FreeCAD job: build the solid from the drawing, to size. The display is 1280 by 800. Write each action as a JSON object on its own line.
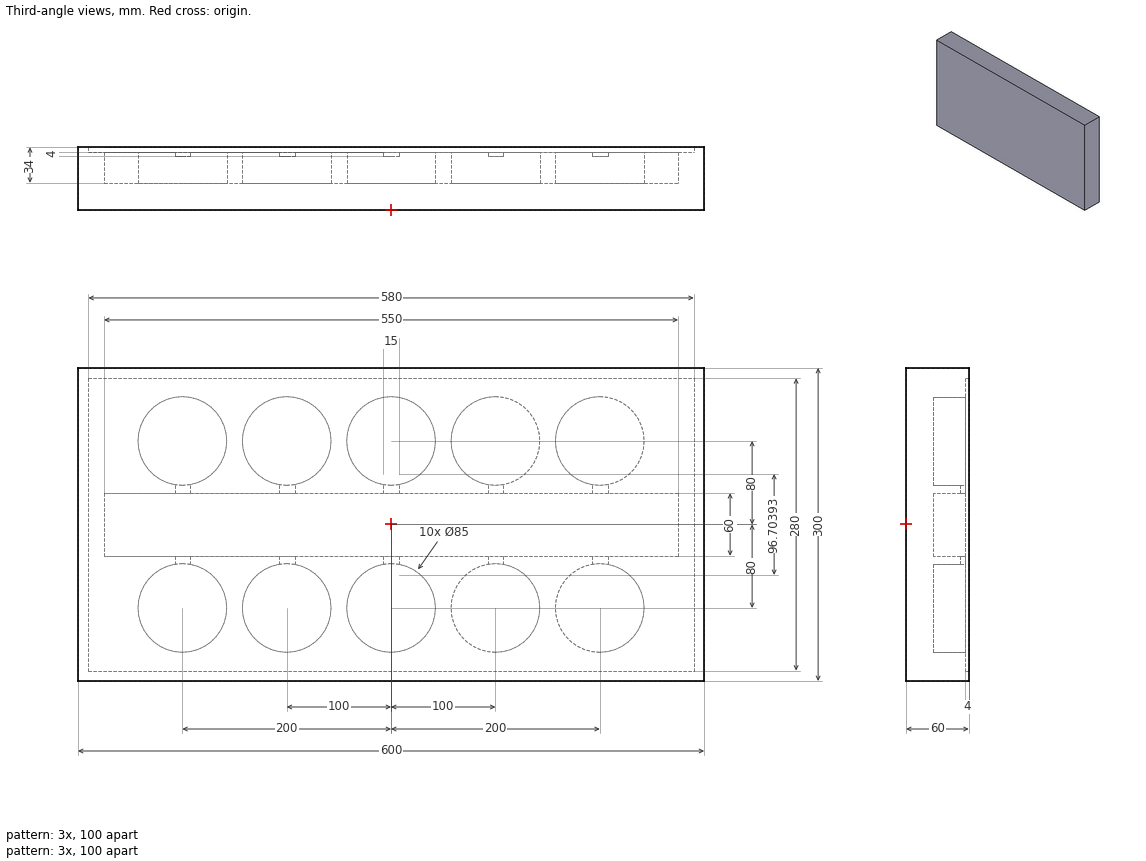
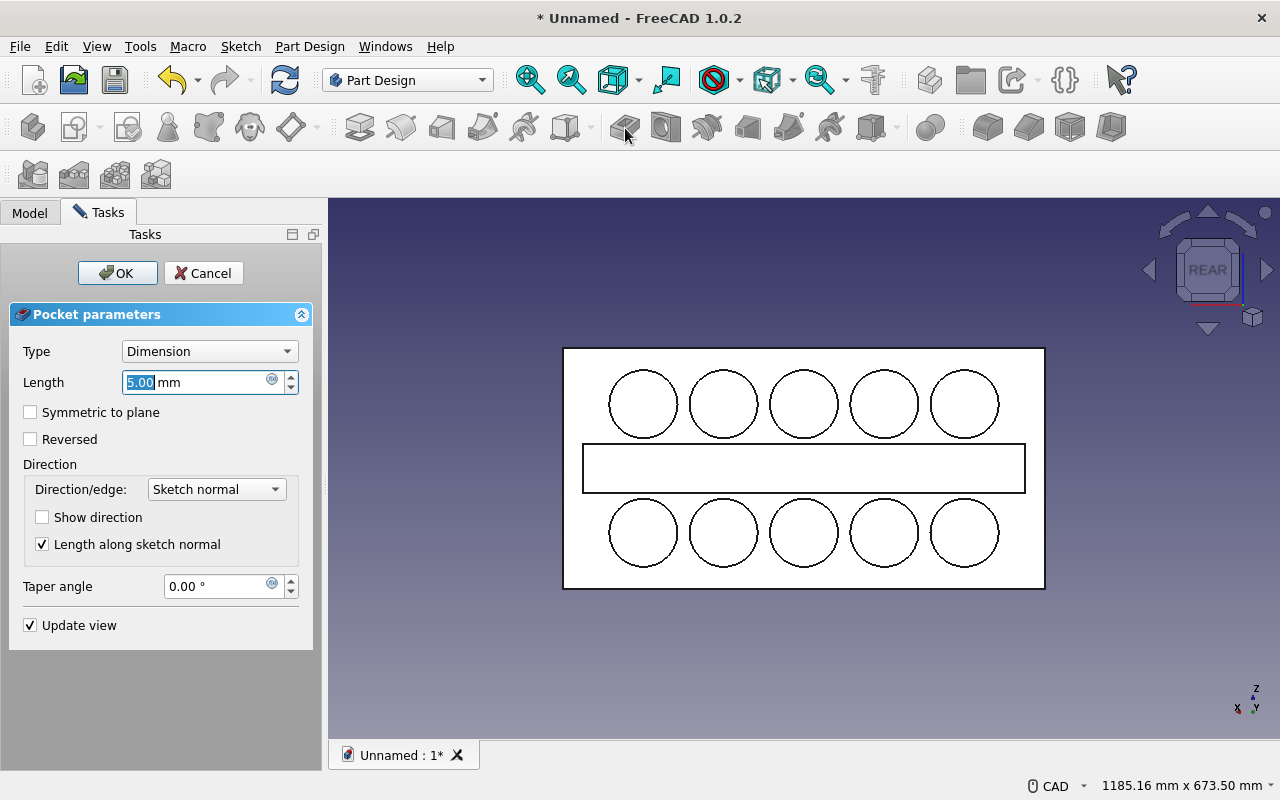
{"action": "type", "text": "34"}
{"action": "key", "text": "Tab"}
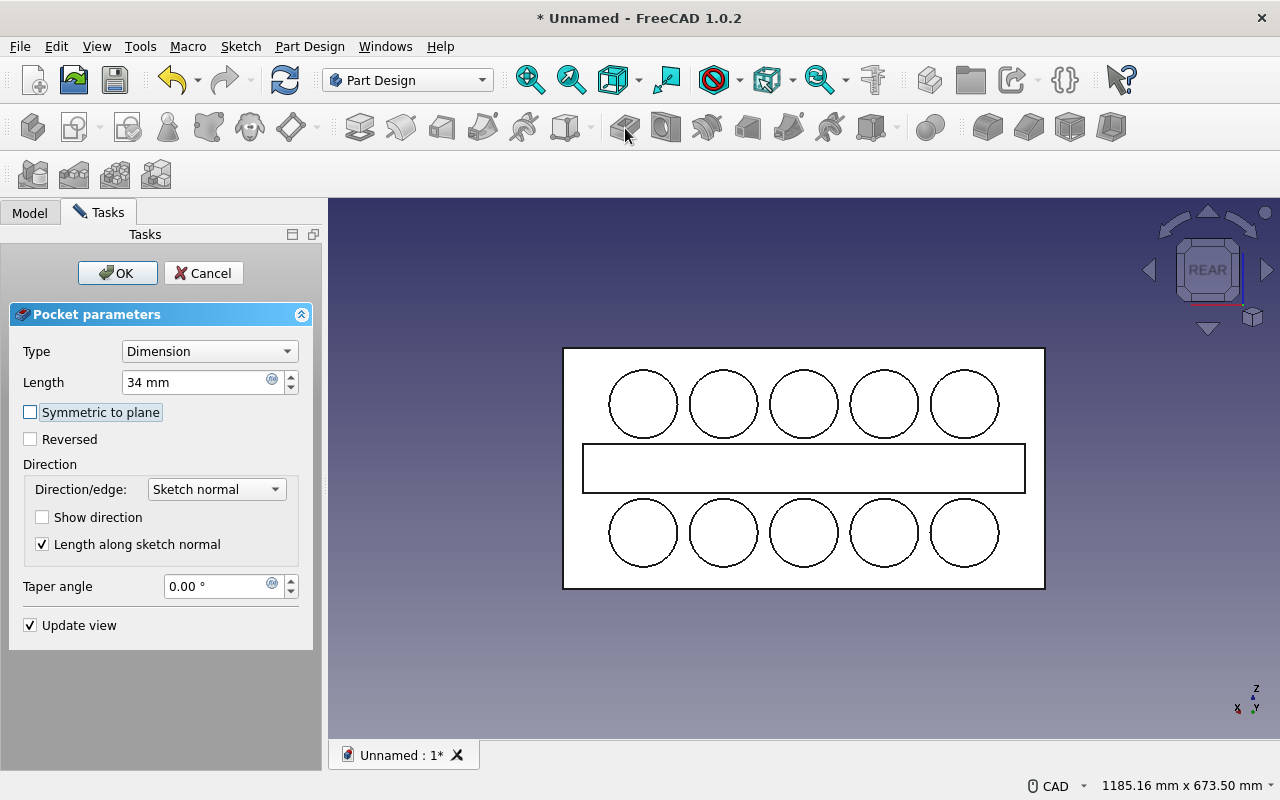
{"action": "left_click", "coordinate": [118, 273]}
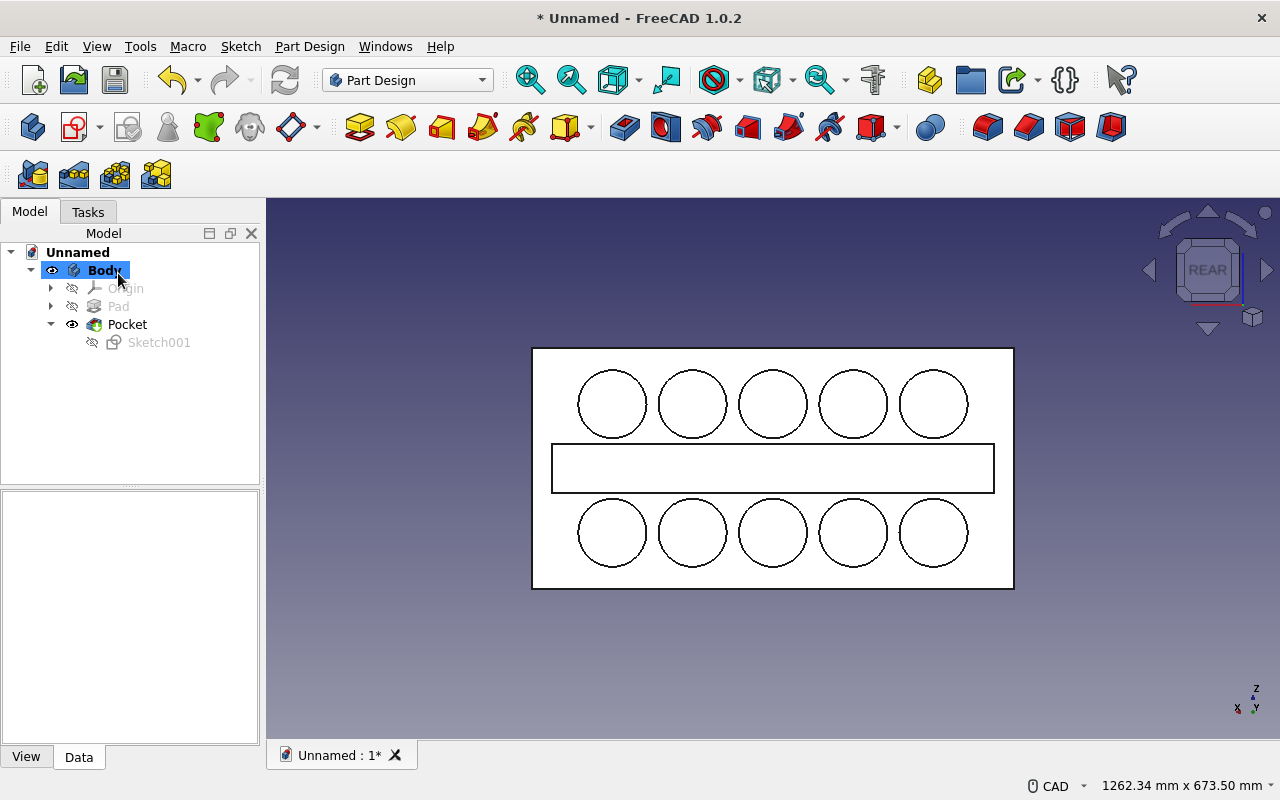
{"action": "left_click", "coordinate": [566, 364]}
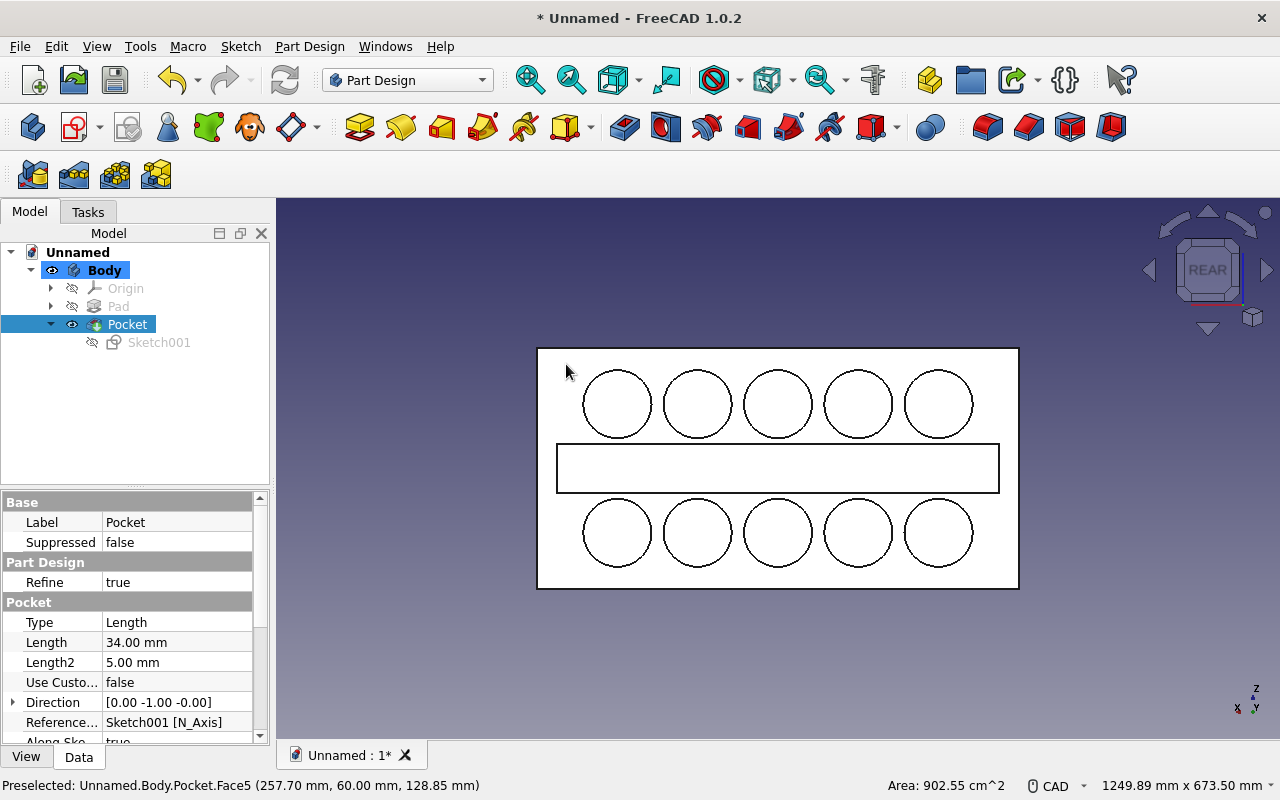
{"action": "left_click", "coordinate": [74, 128]}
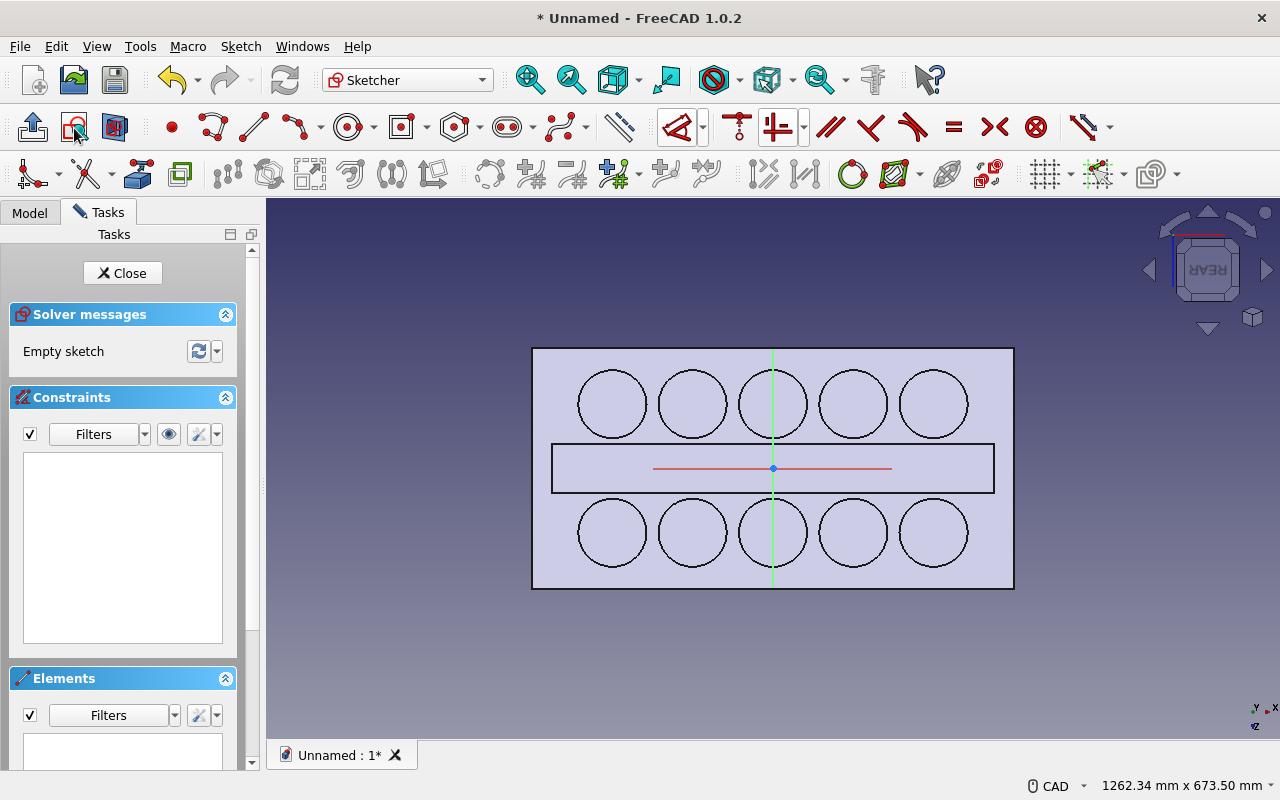
{"action": "left_click", "coordinate": [400, 128]}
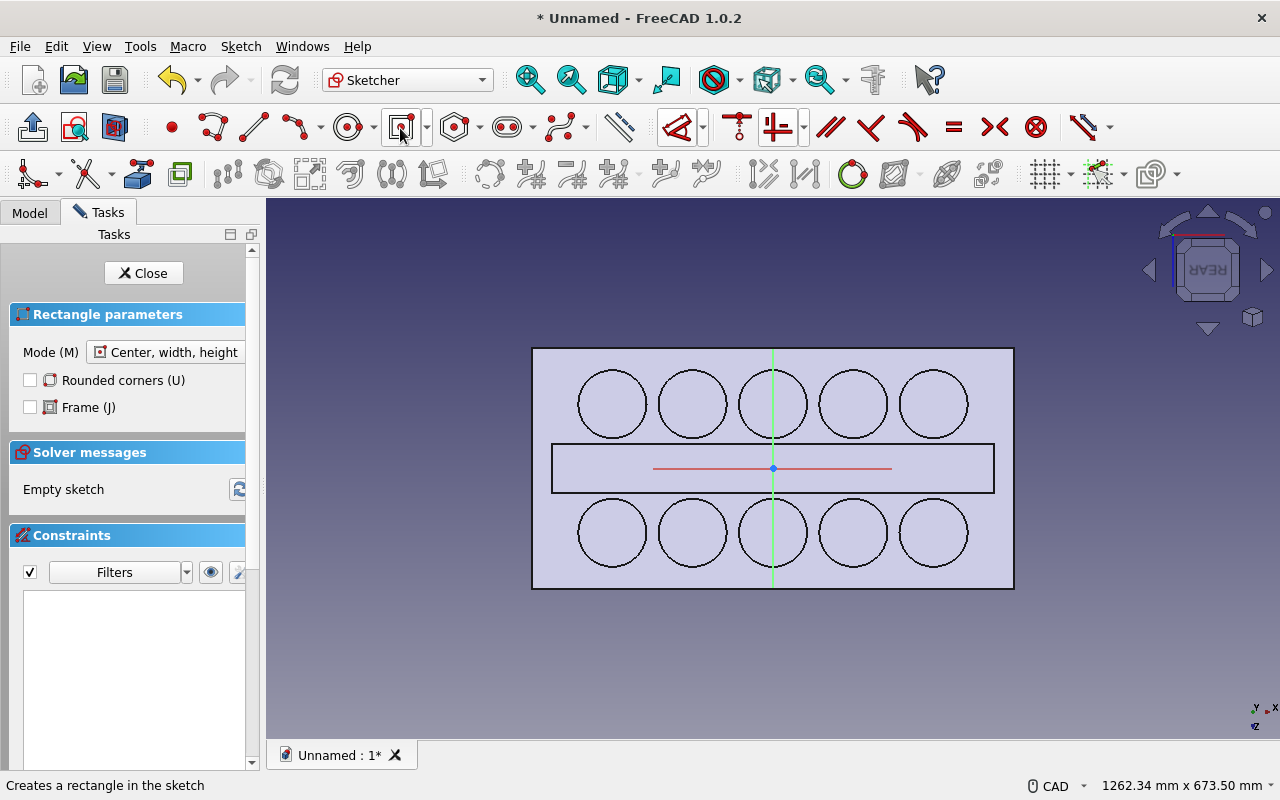
{"action": "left_click", "coordinate": [773, 468]}
{"action": "mouse_move", "coordinate": [1006, 356]}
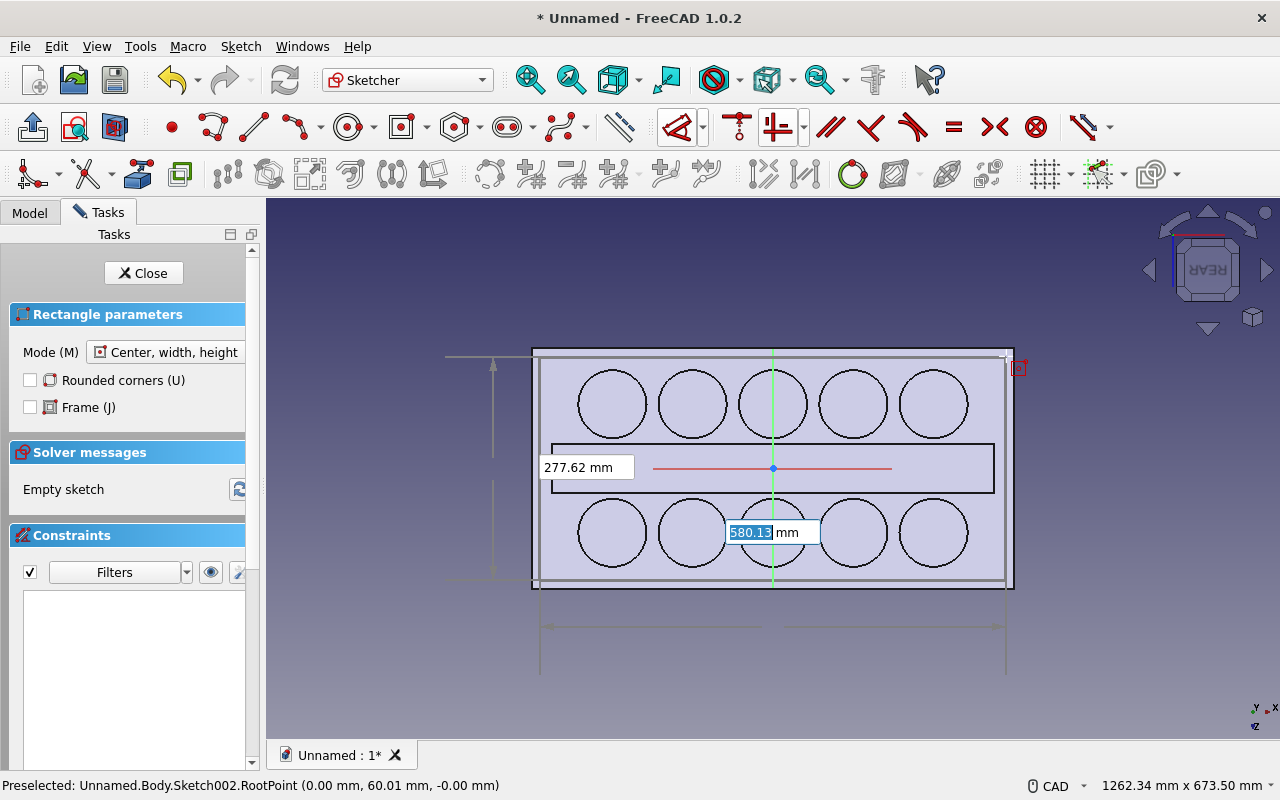
{"action": "type", "text": "580"}
{"action": "key", "text": "Tab"}
{"action": "type", "text": "280"}
{"action": "key", "text": "Return"}
{"action": "key", "text": "Escape"}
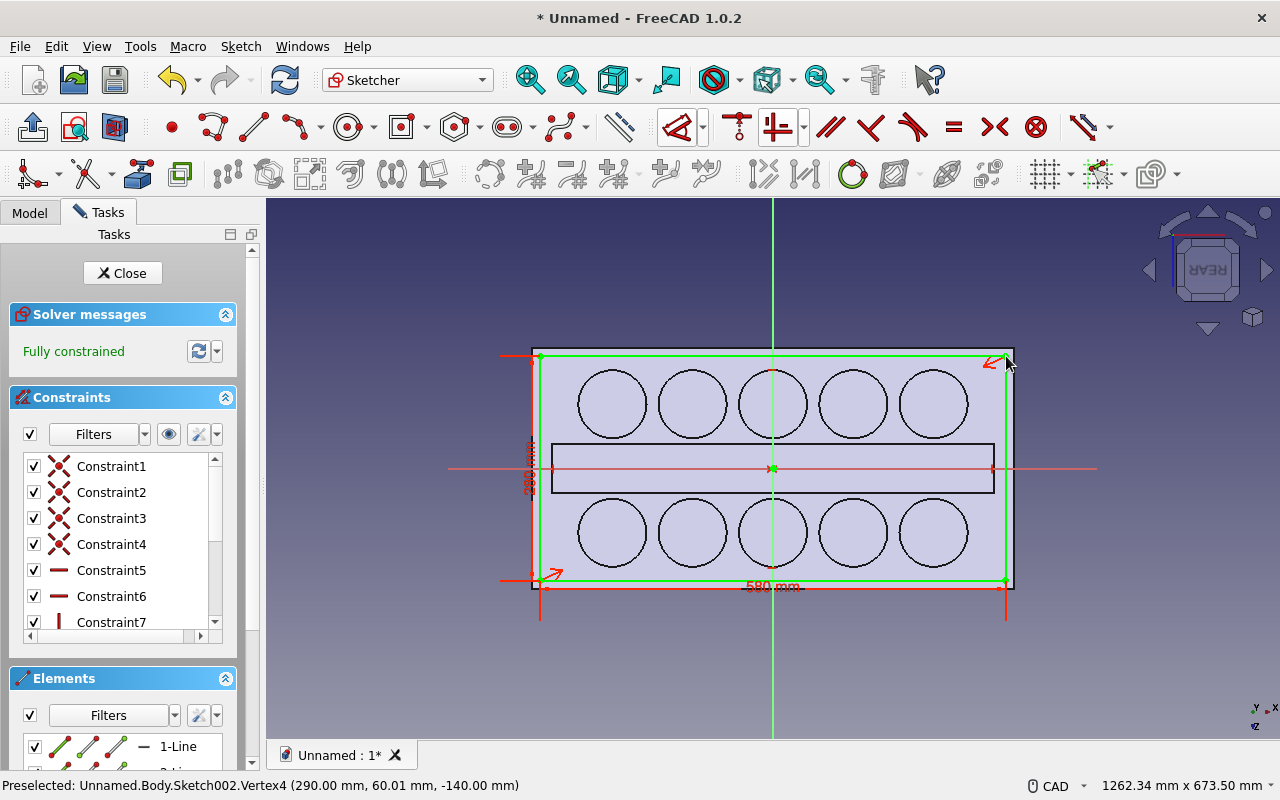
{"action": "left_click", "coordinate": [123, 273]}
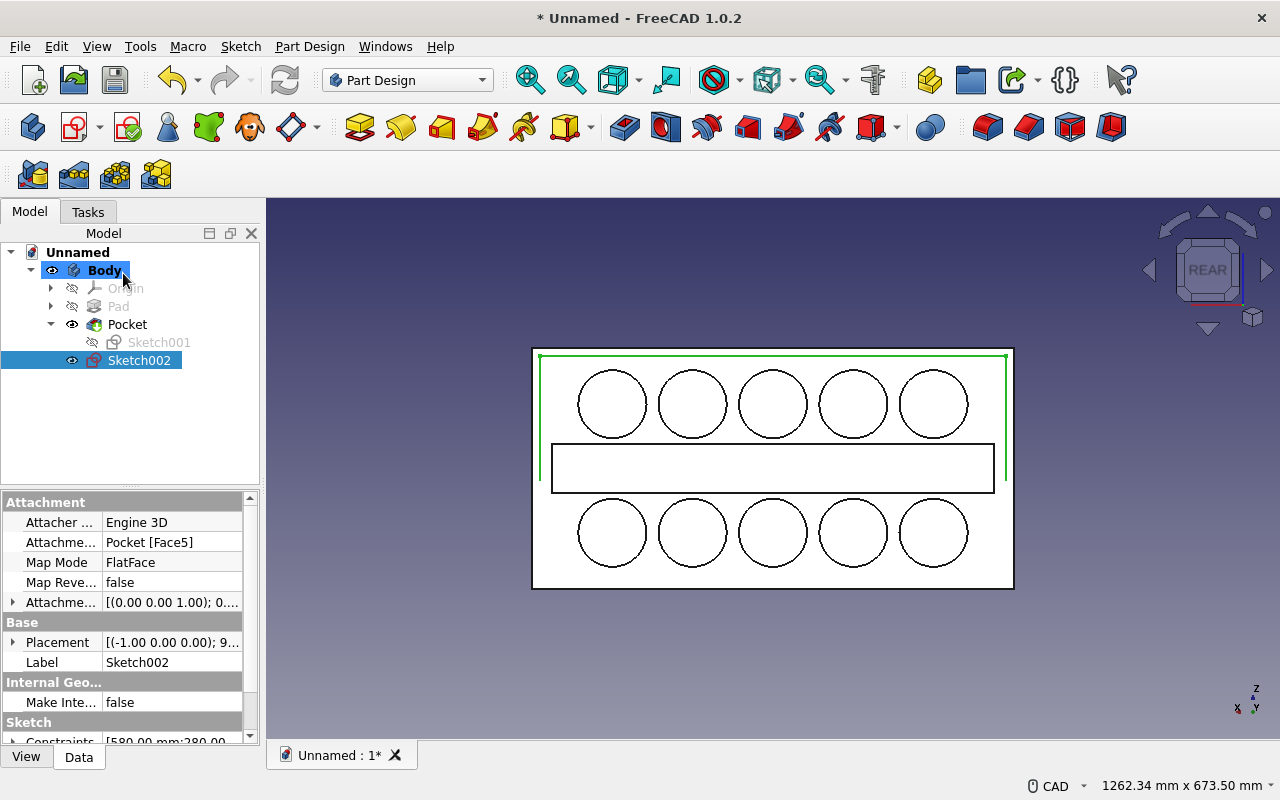
{"action": "left_click", "coordinate": [625, 128]}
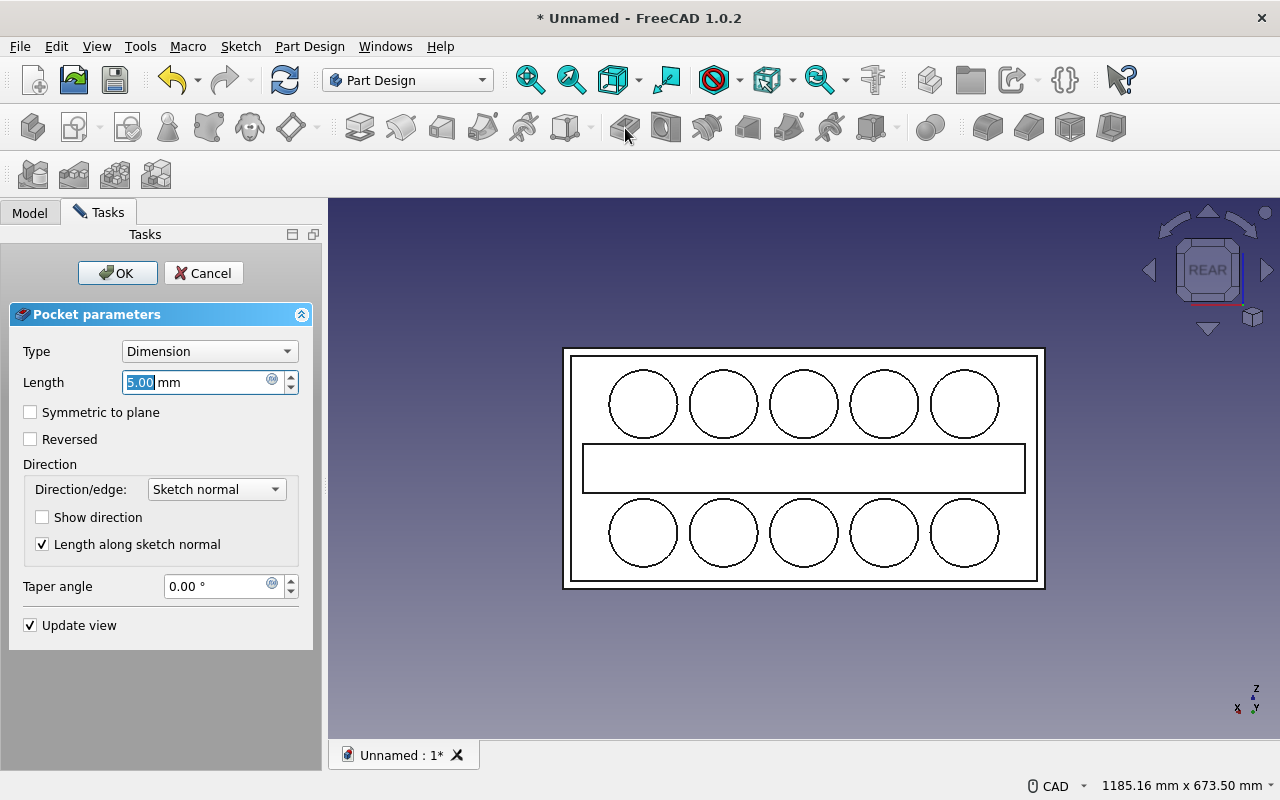
{"action": "type", "text": "4"}
{"action": "key", "text": "Tab"}